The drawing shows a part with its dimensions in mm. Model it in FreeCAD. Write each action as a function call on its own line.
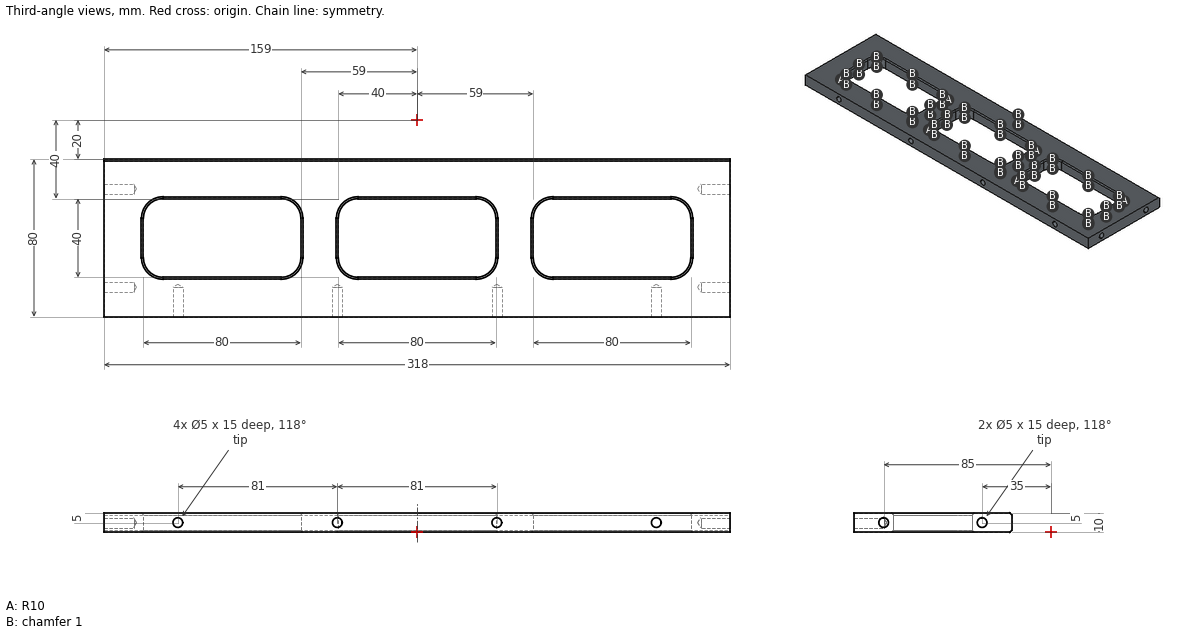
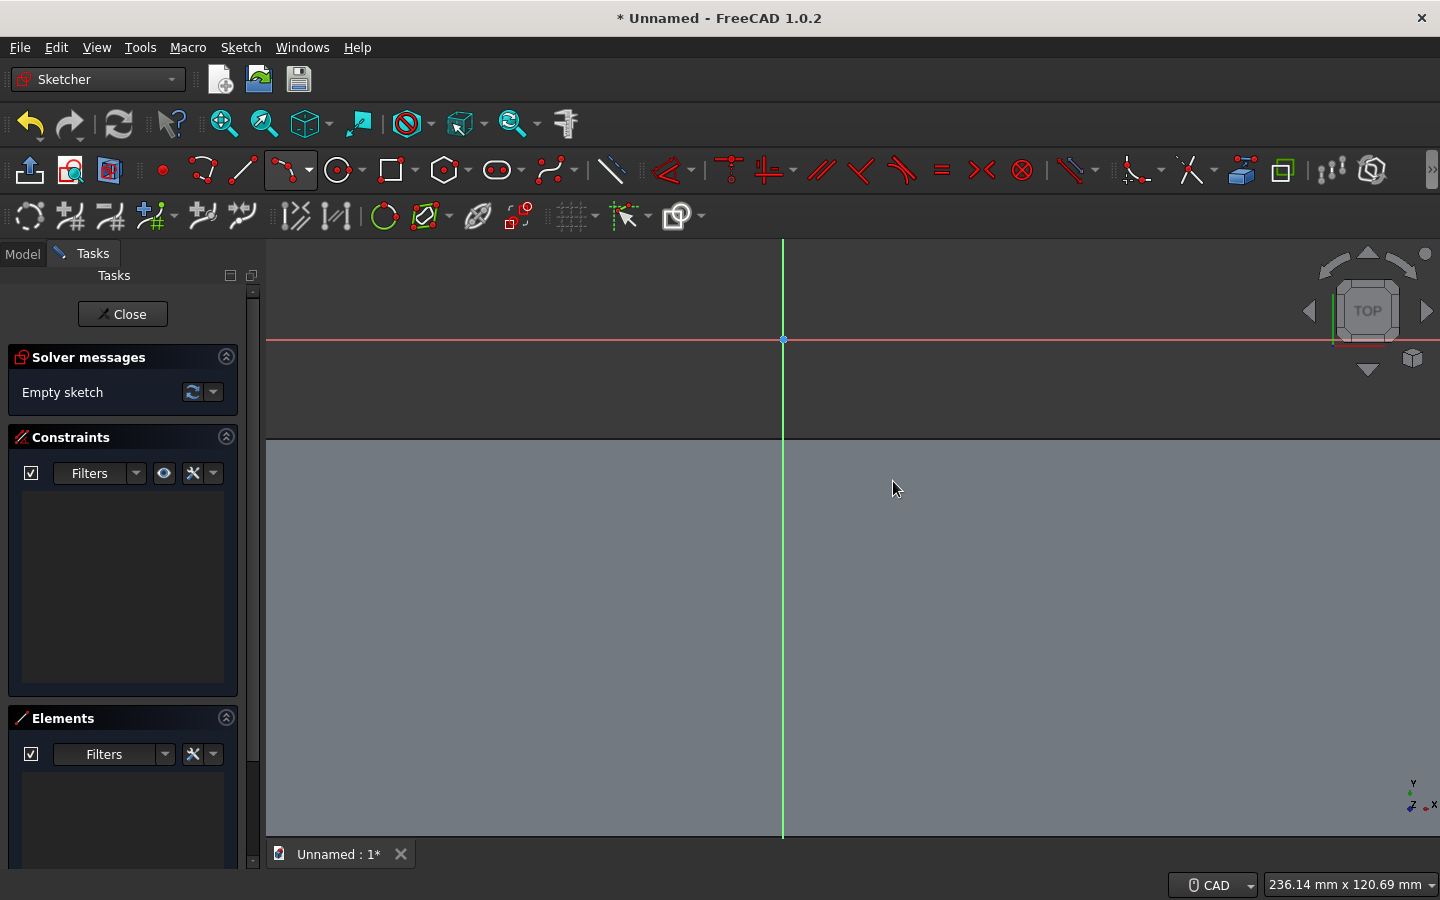
key(g)
key(r)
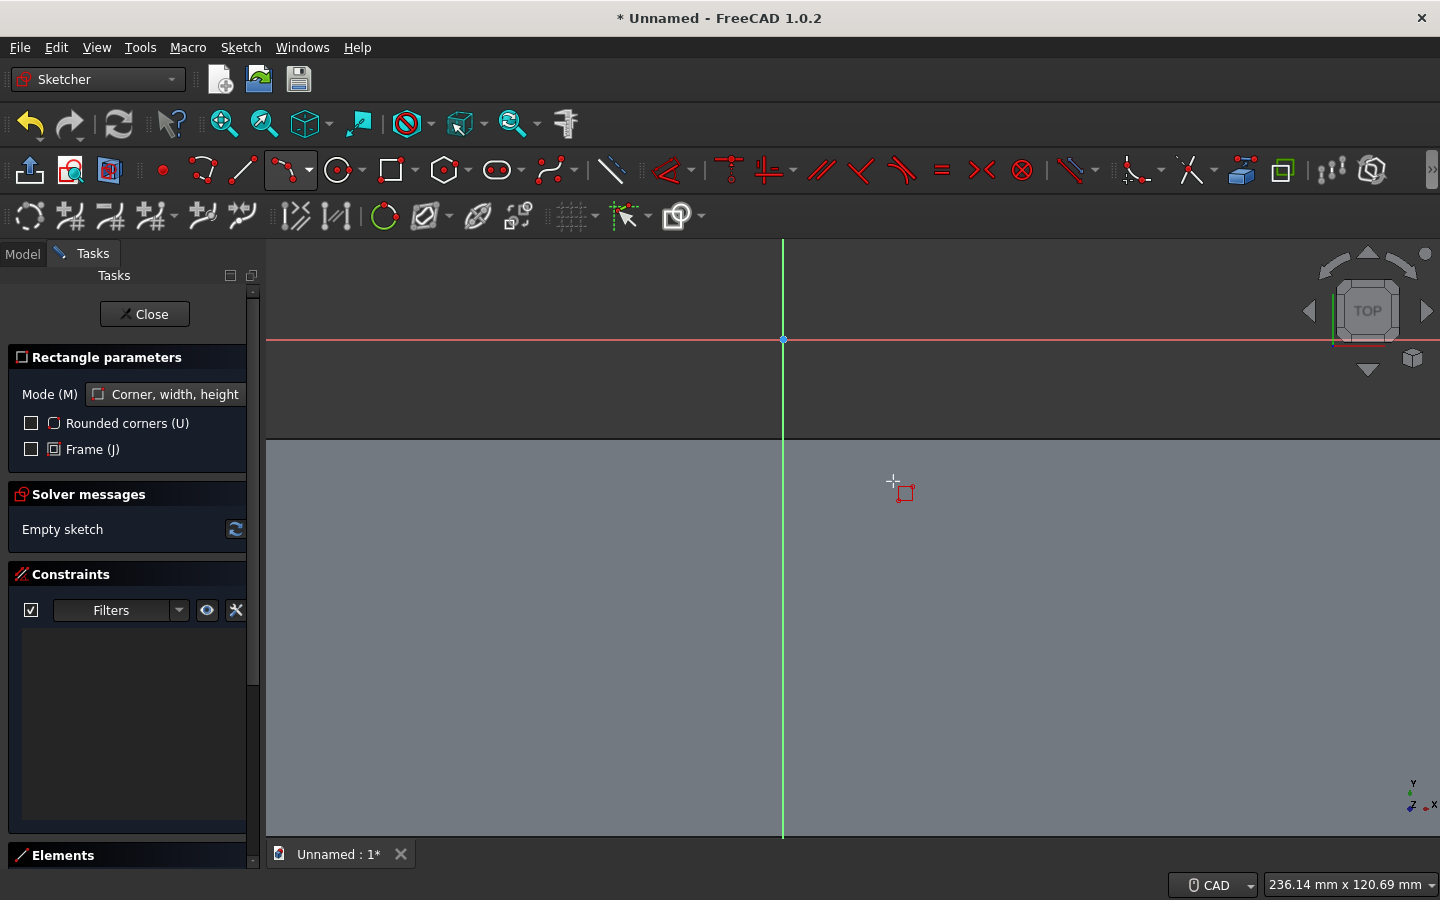
click(584, 539)
click(982, 737)
key(Escape)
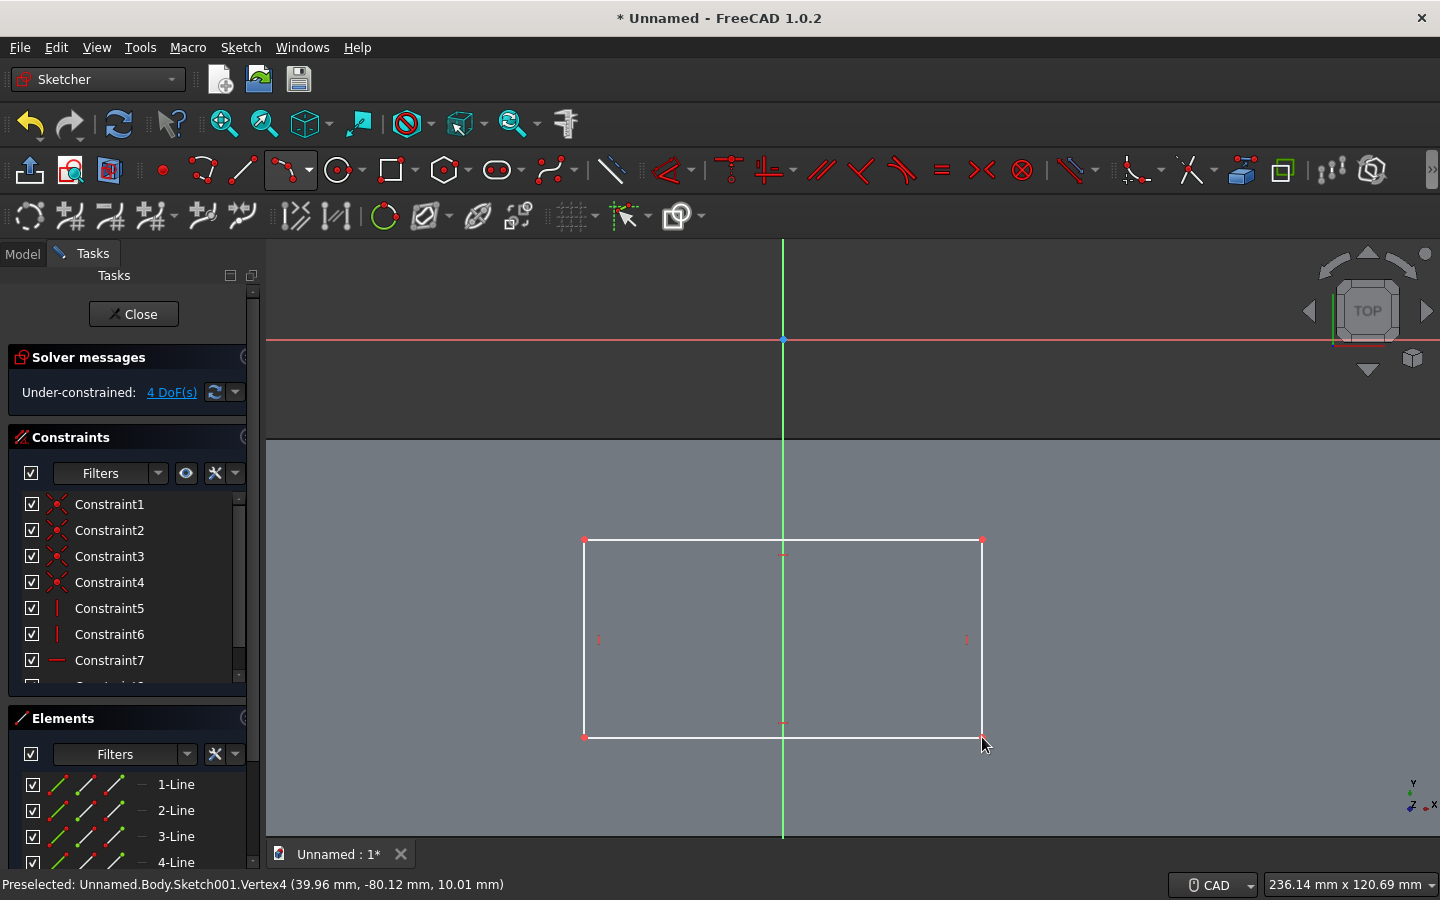
click(666, 170)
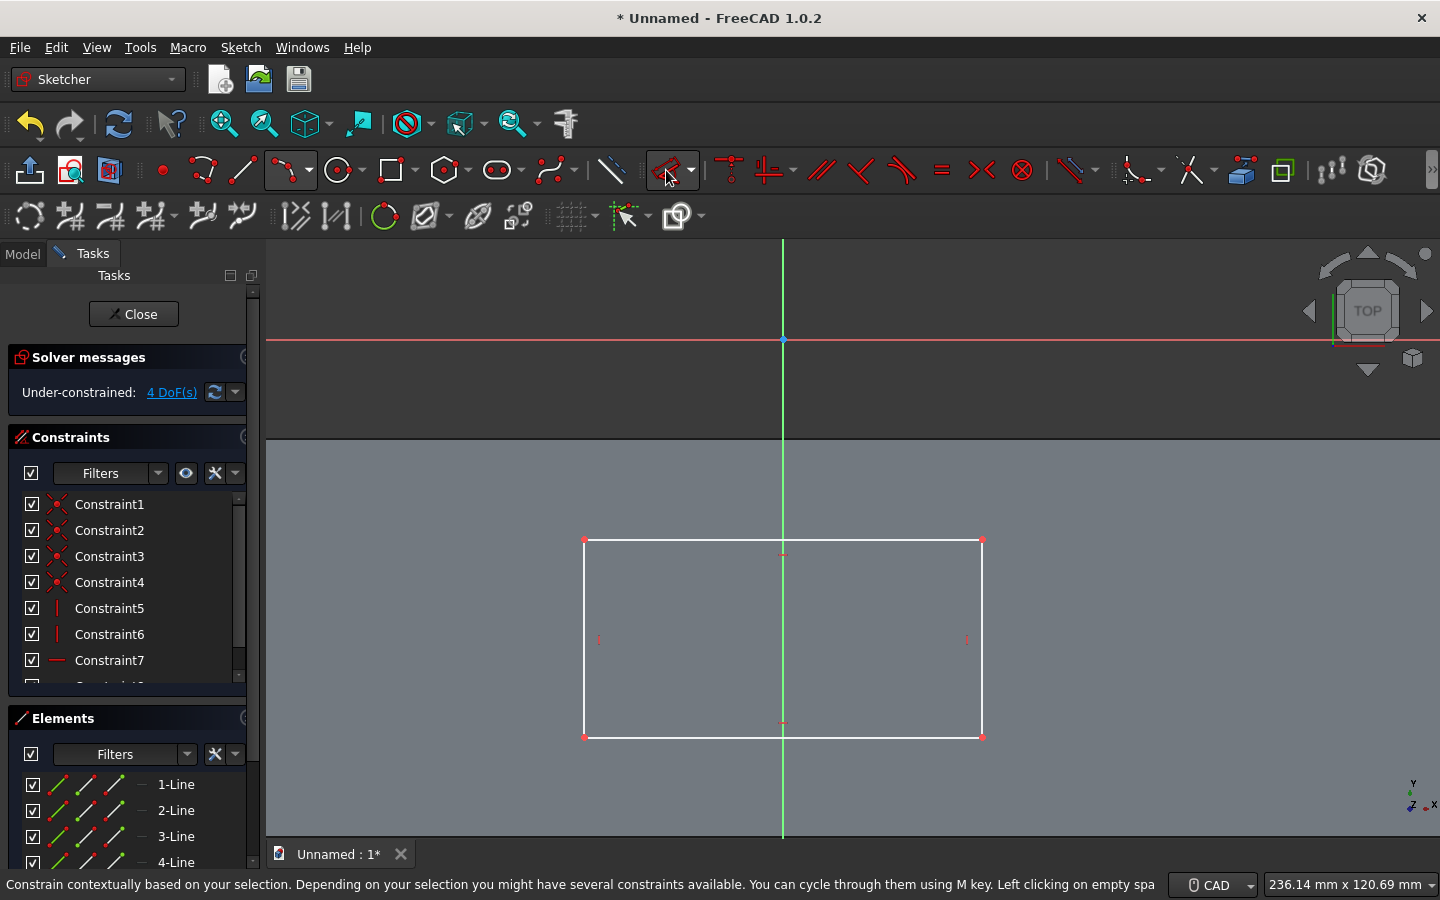
click(584, 599)
click(550, 639)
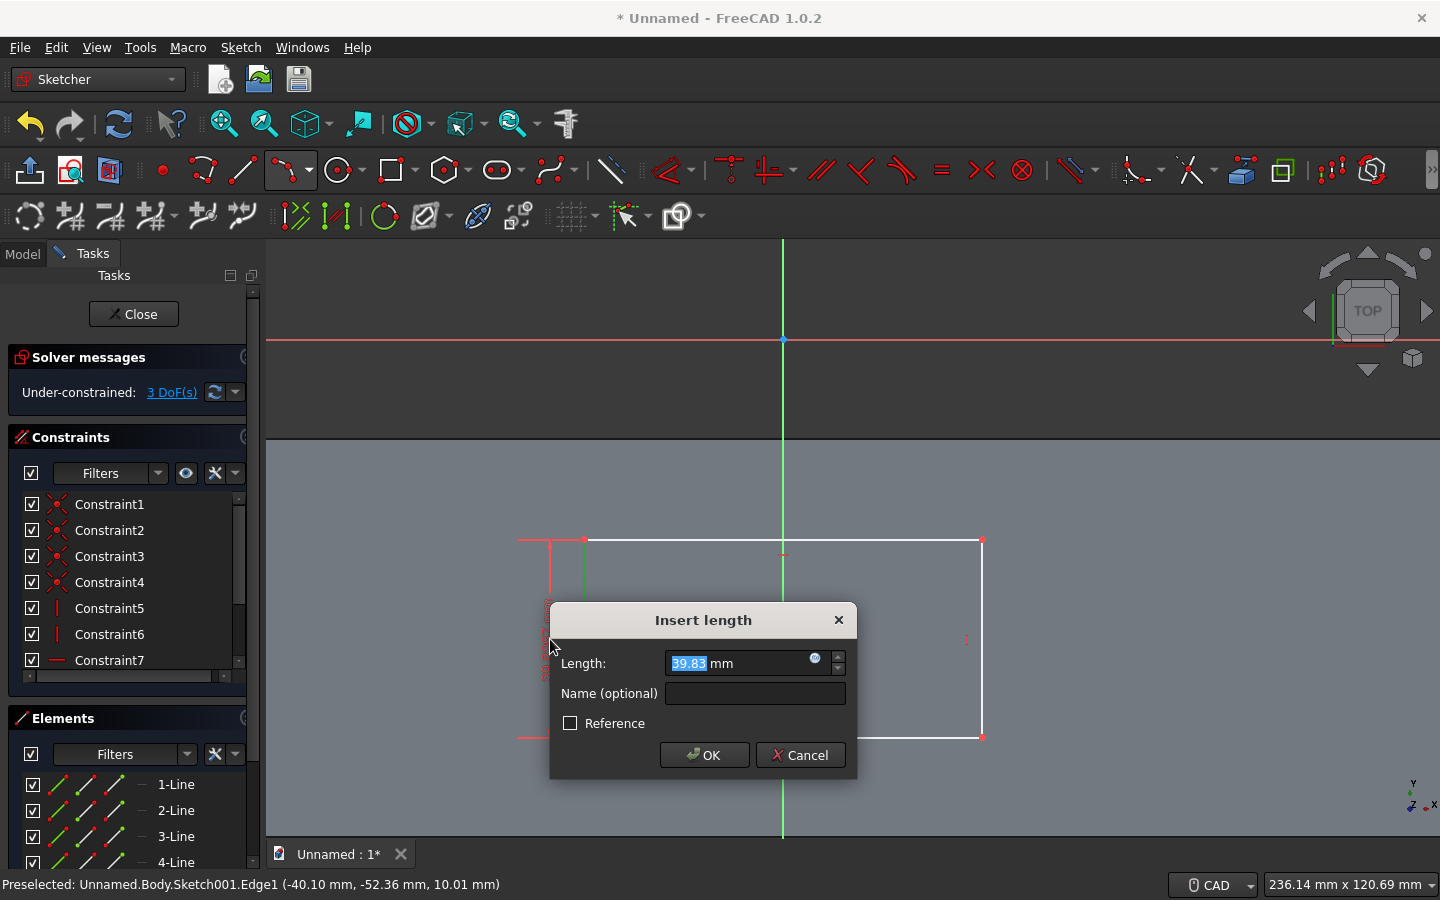
text(40)
key(Return)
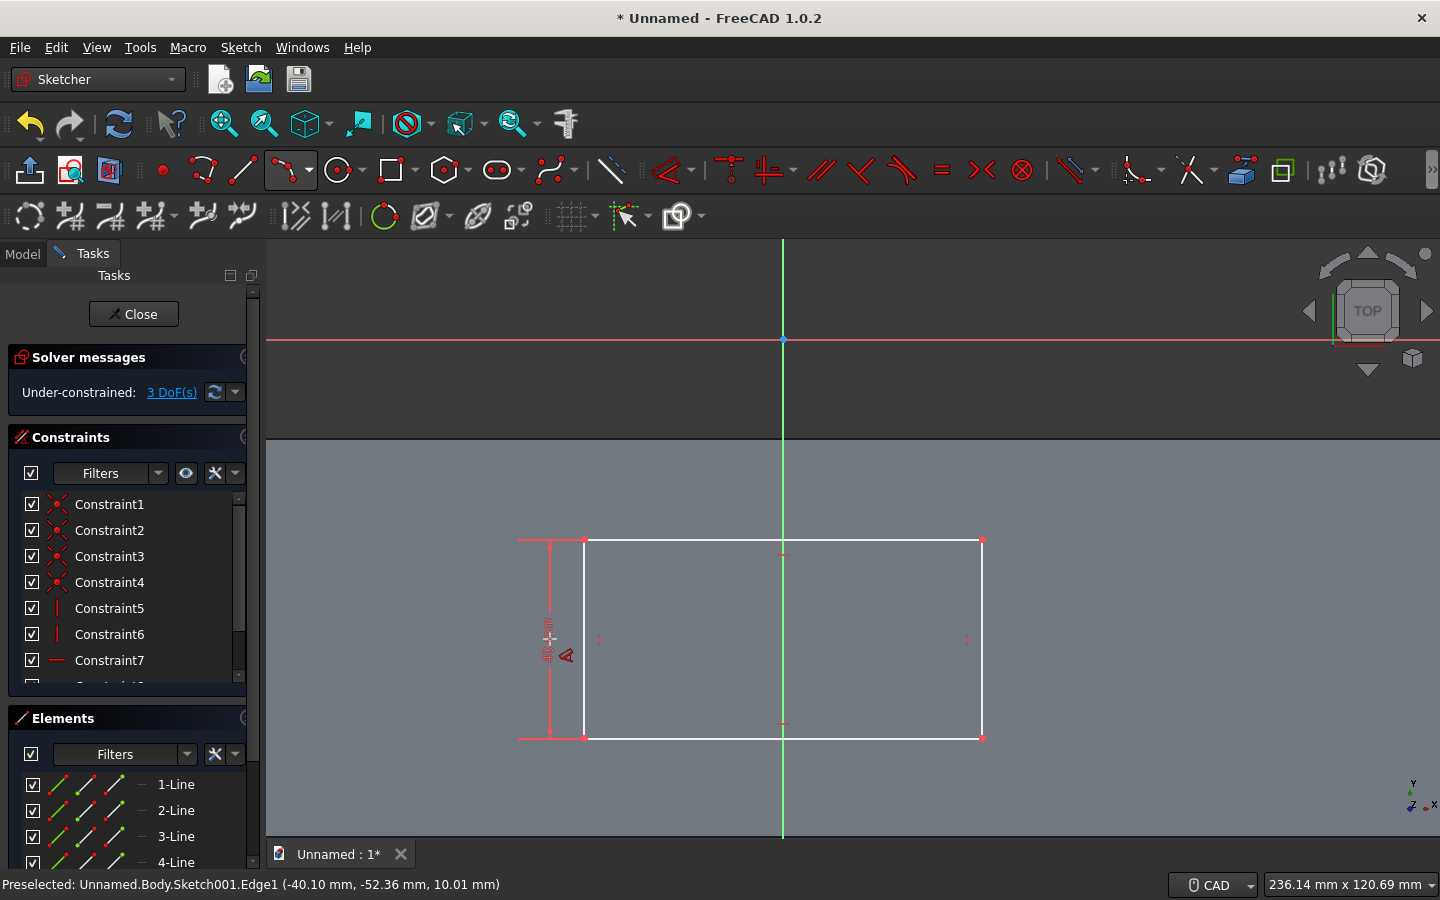
click(703, 739)
click(691, 773)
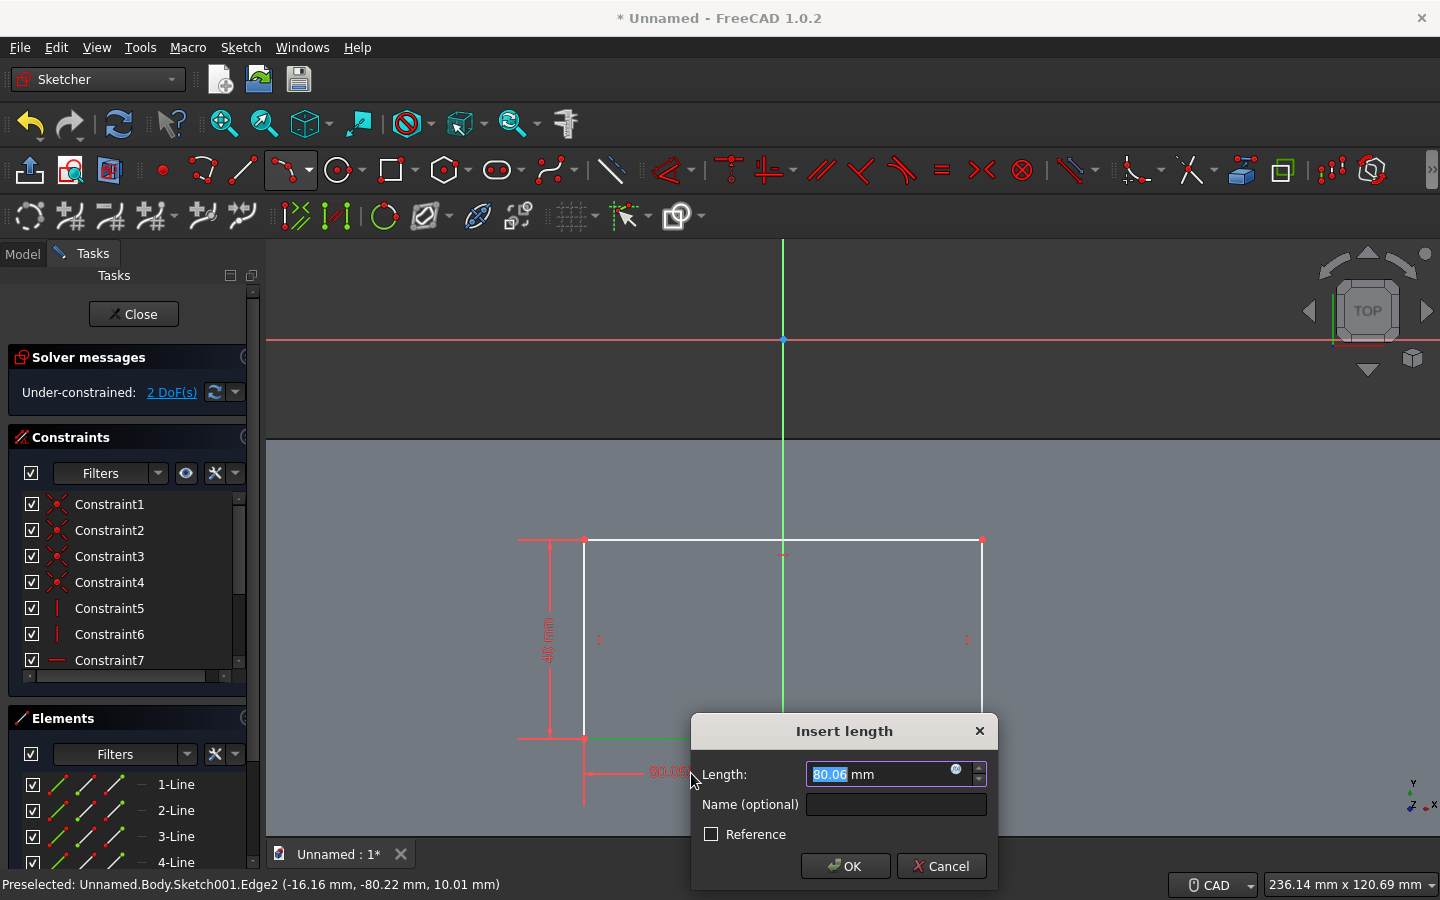
text(80)
key(Return)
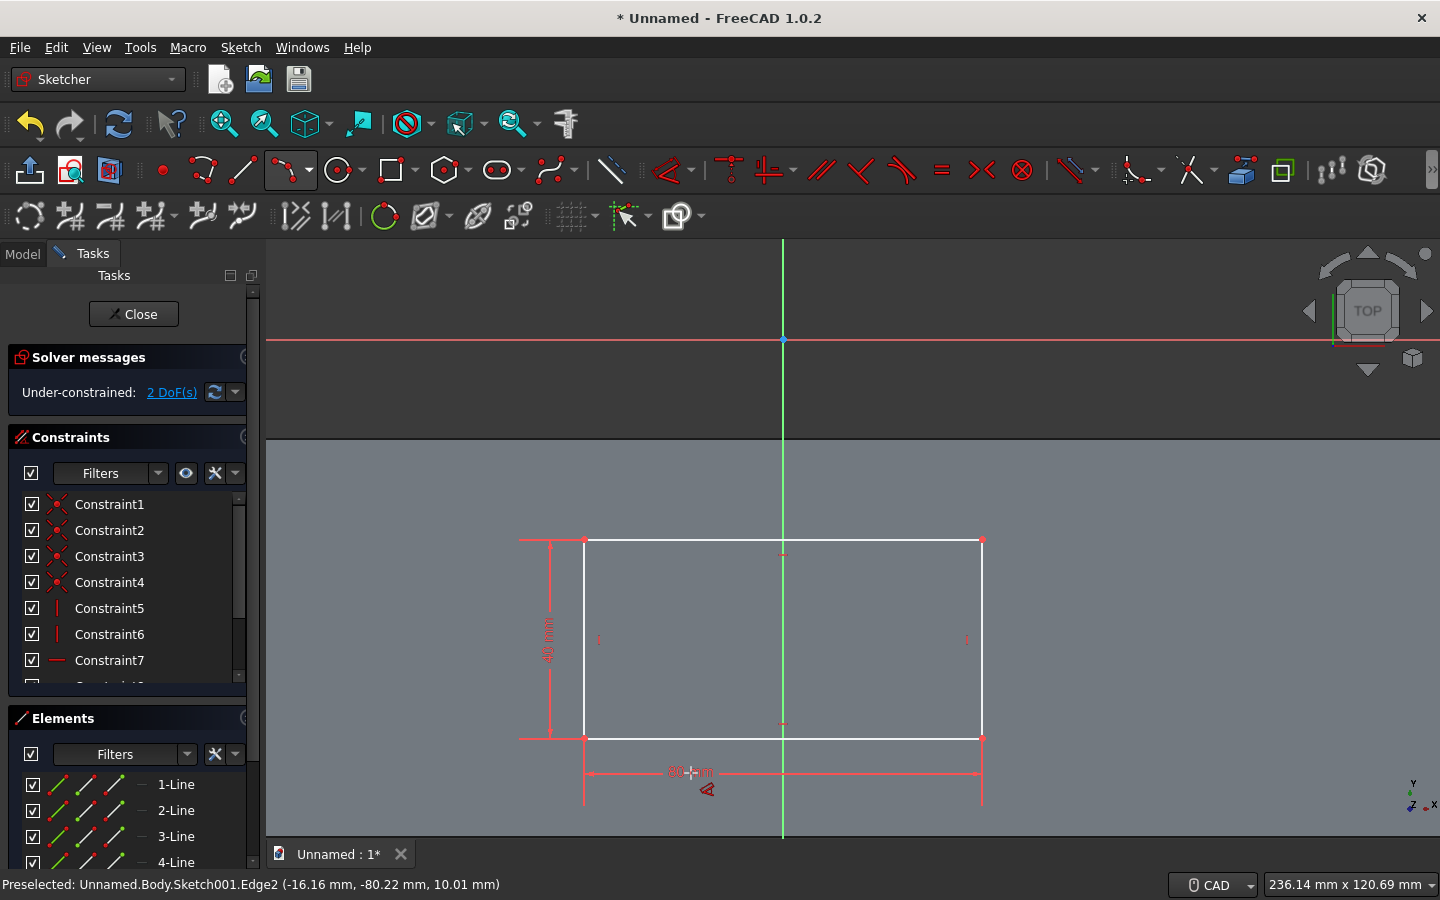
click(584, 540)
click(684, 306)